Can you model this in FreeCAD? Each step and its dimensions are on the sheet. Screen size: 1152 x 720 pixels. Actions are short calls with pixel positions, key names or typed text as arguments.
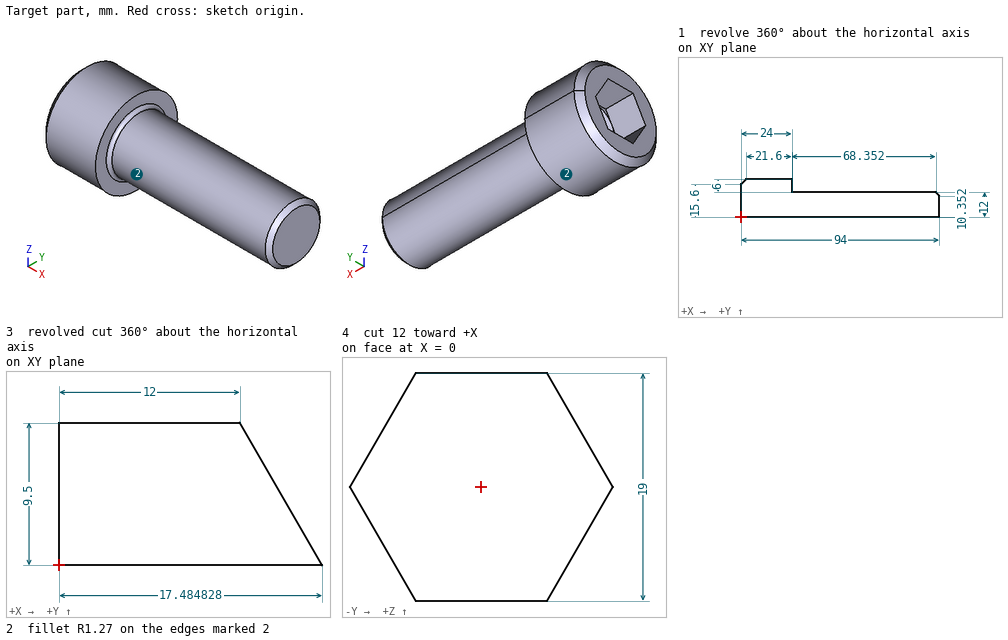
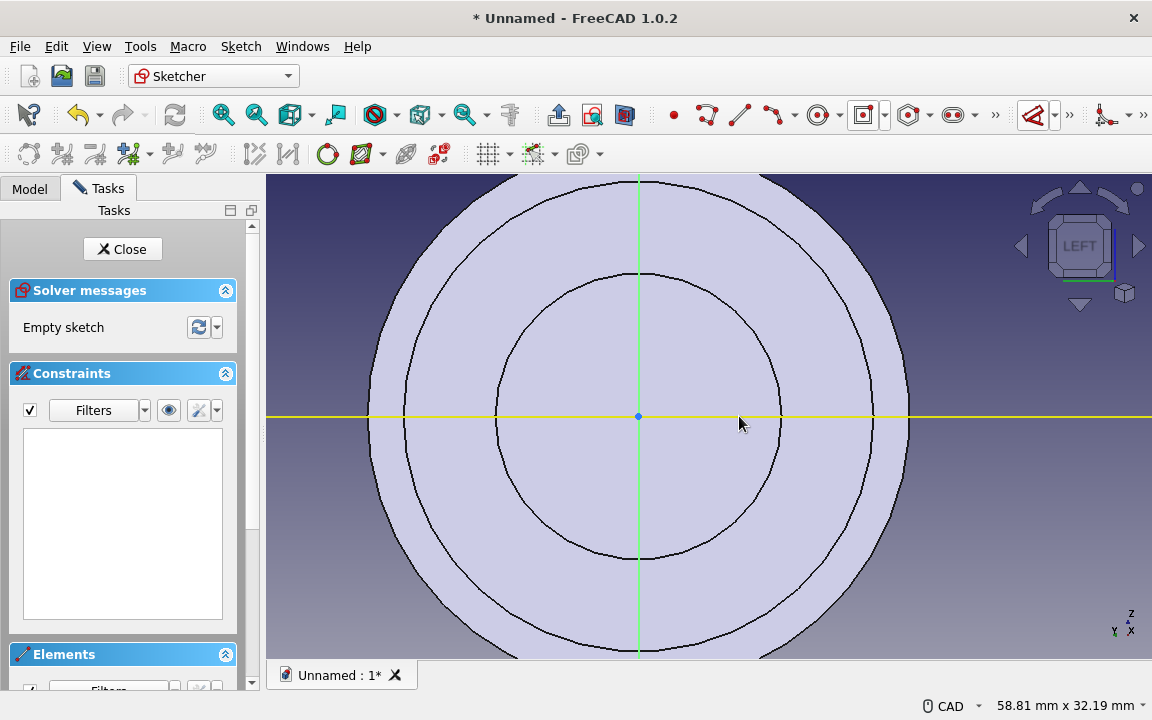
click(908, 116)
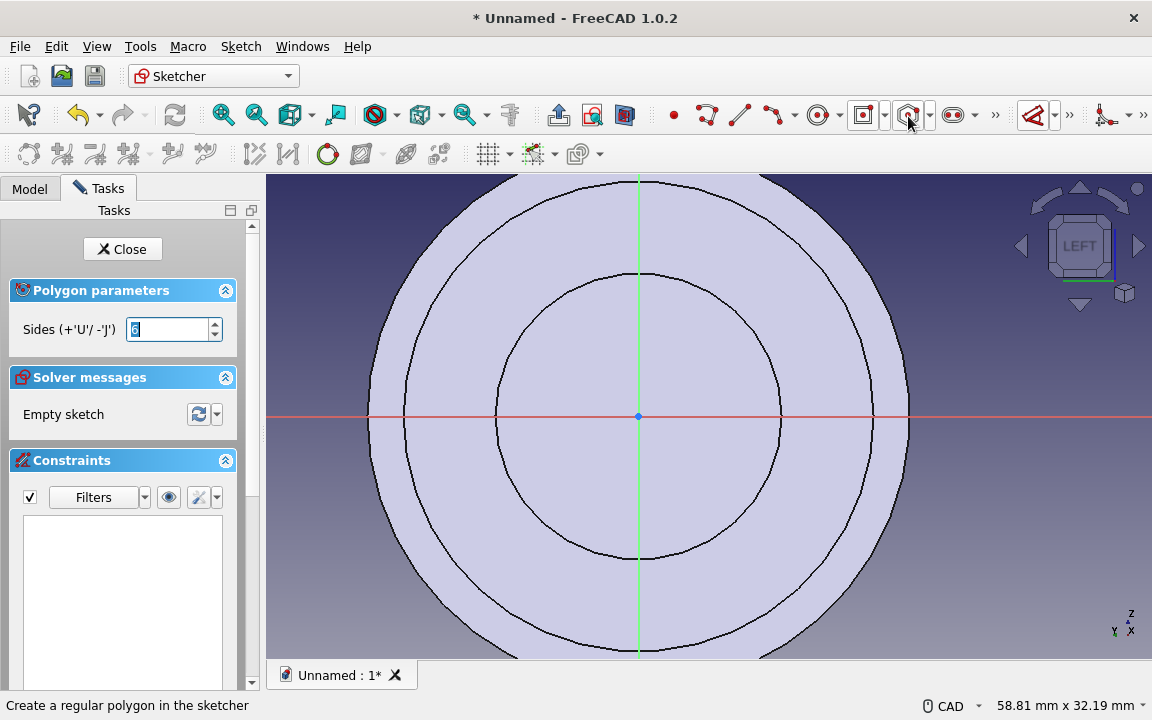
click(639, 416)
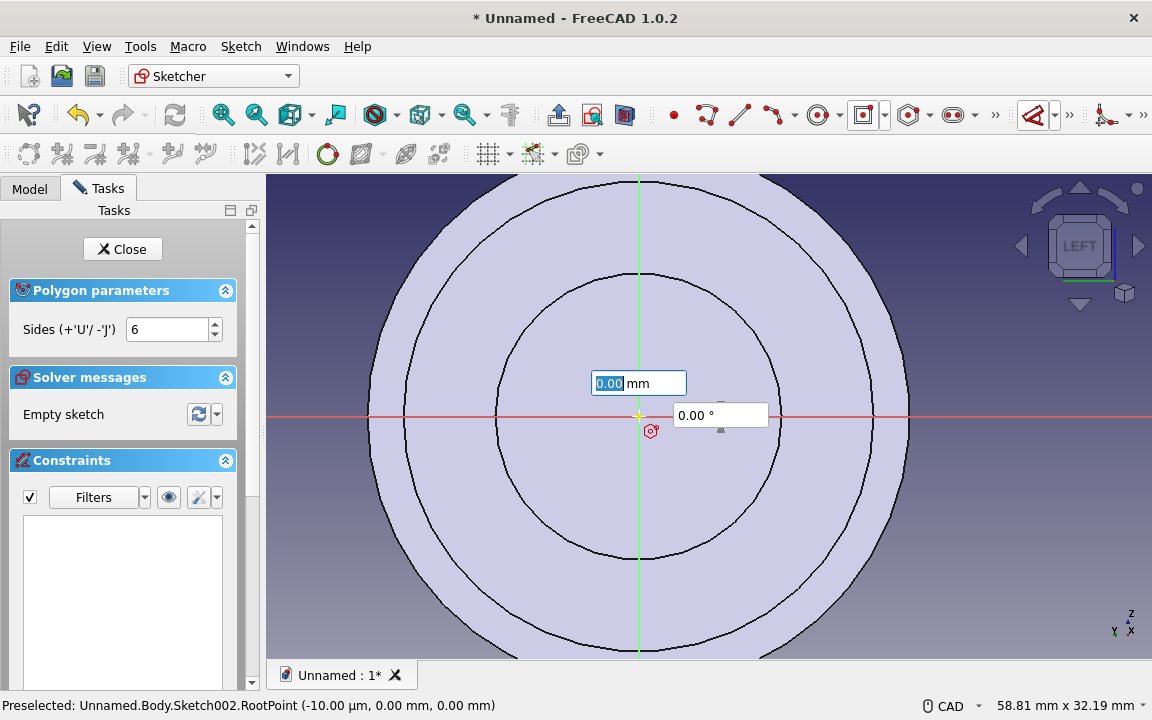
click(473, 416)
right_click(473, 416)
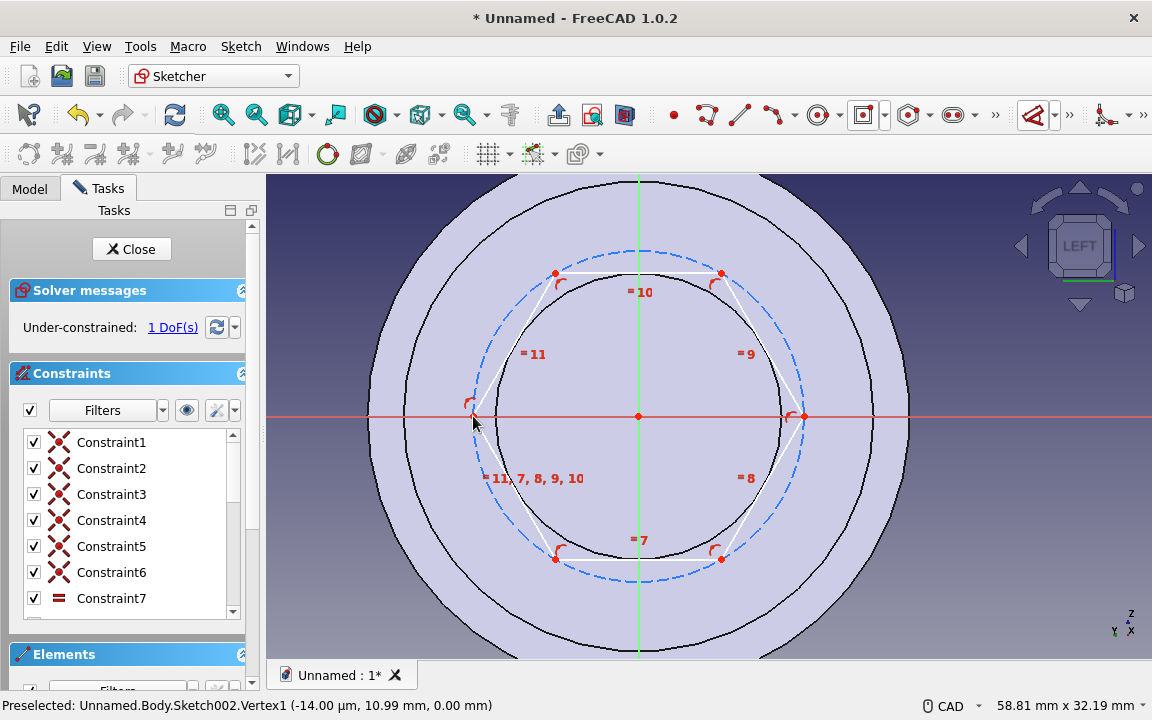
click(721, 560)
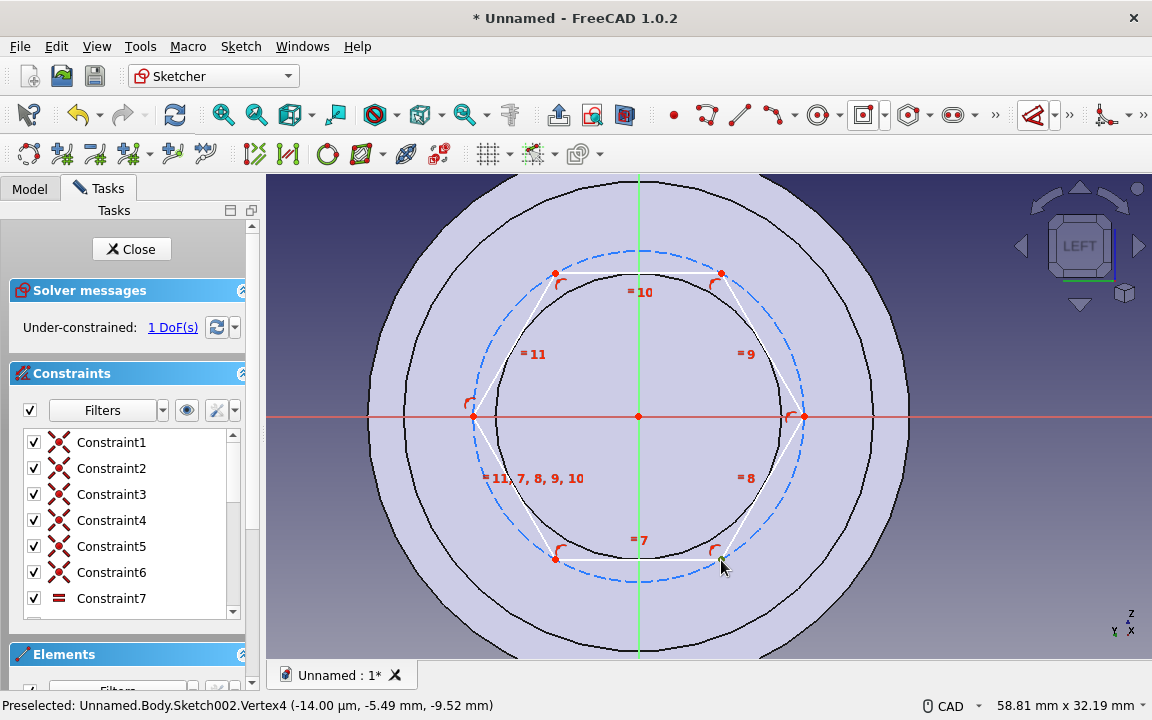
click(556, 273)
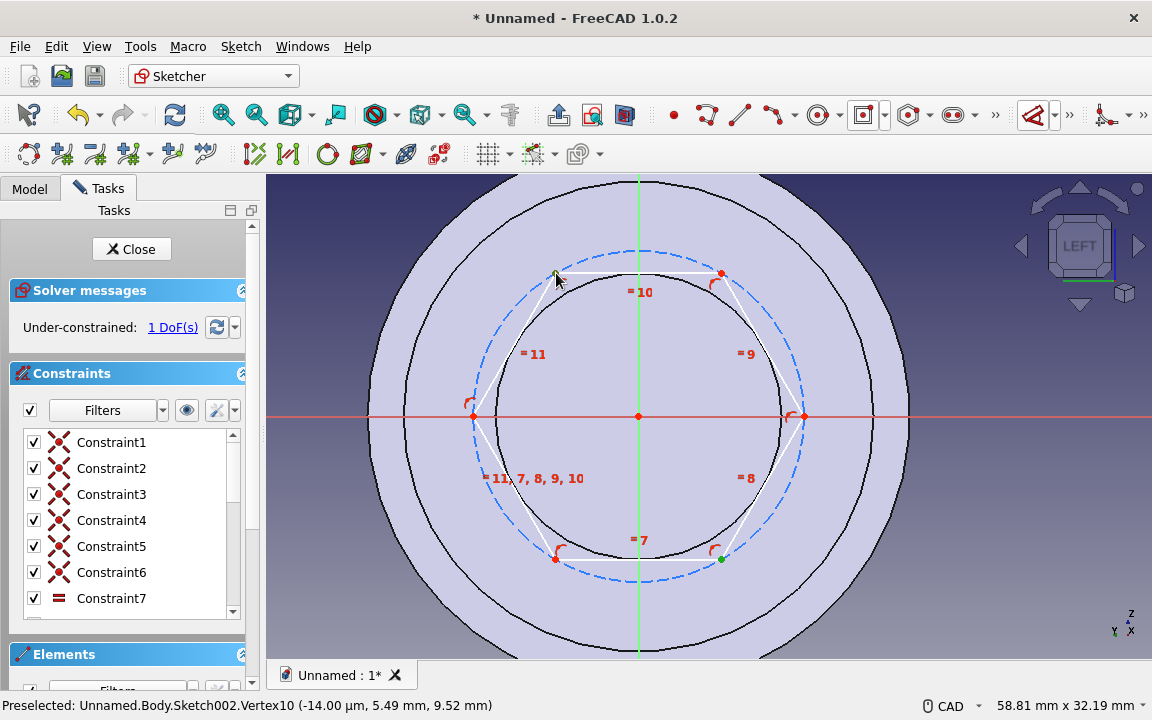
key(i)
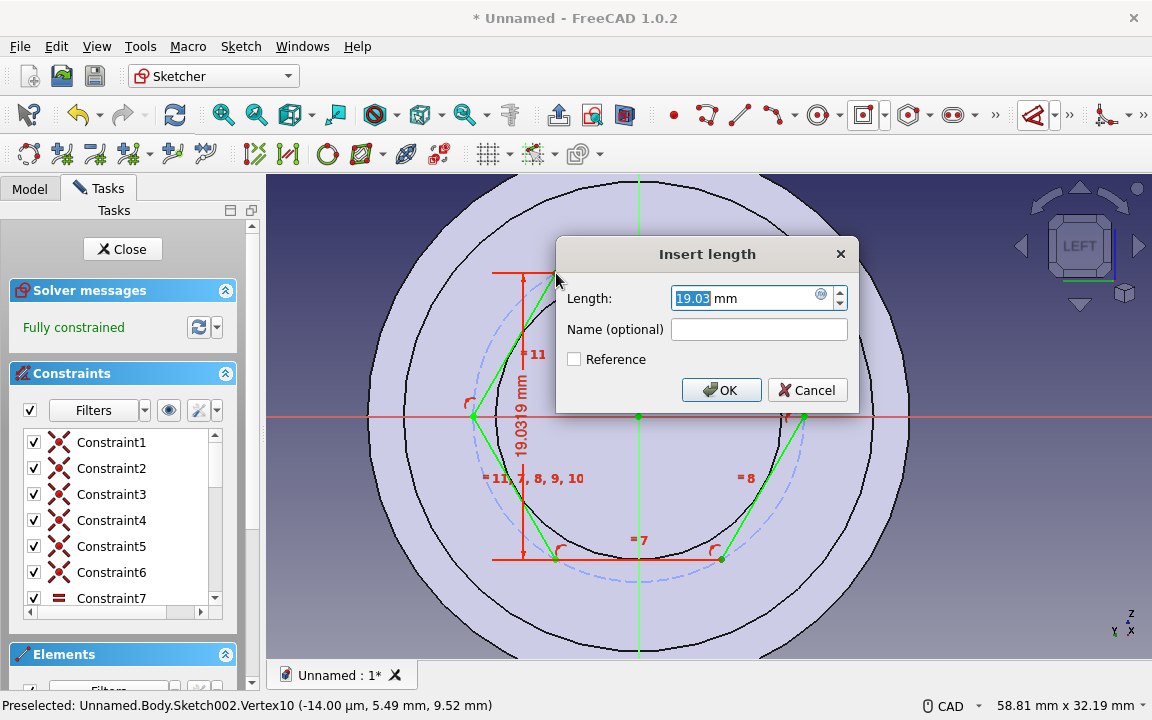
text(19)
key(Return)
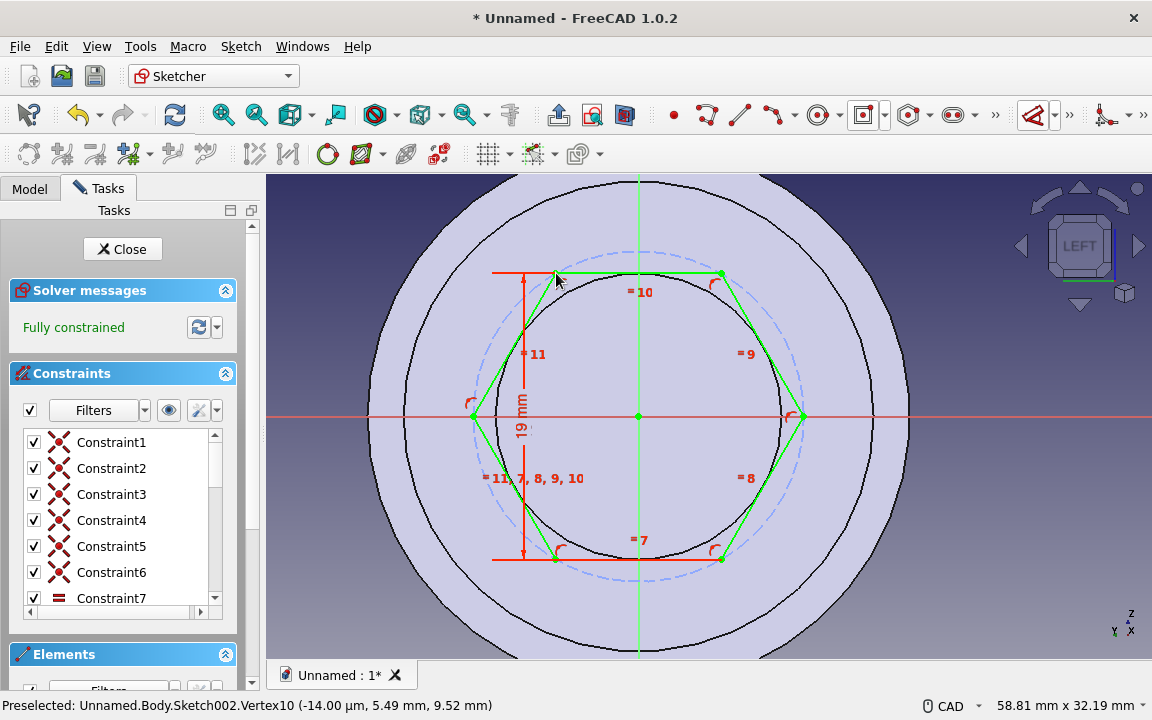
click(123, 249)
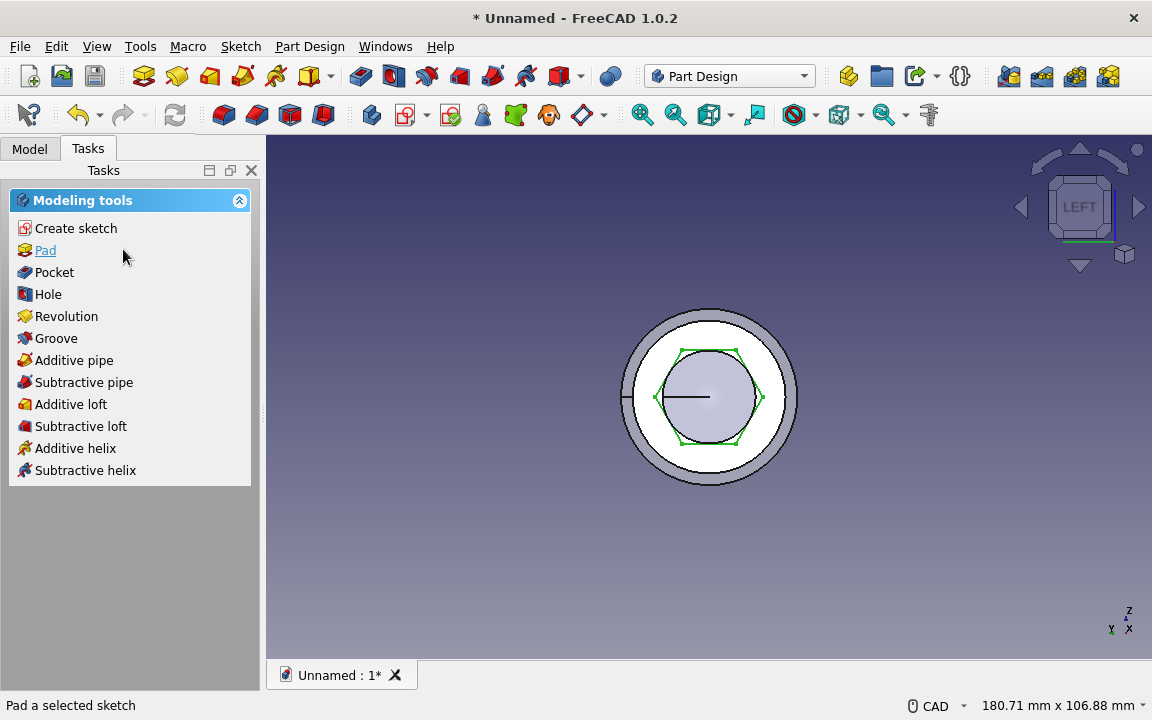
click(361, 76)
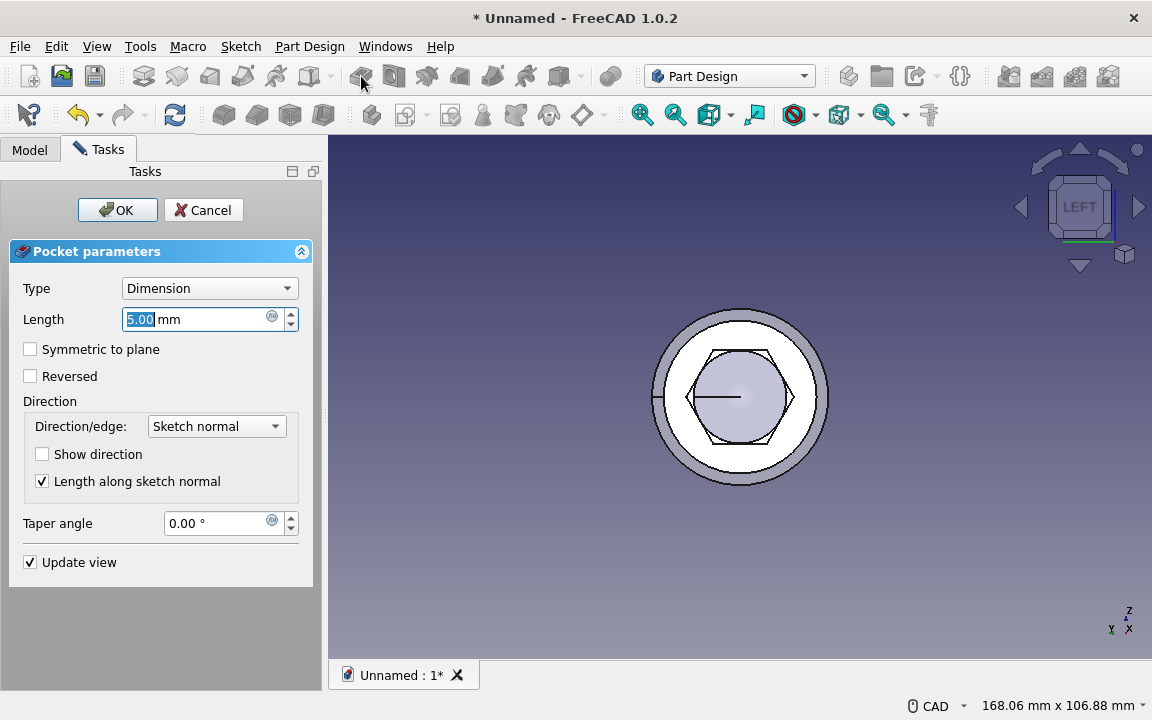
text(12)
key(Tab)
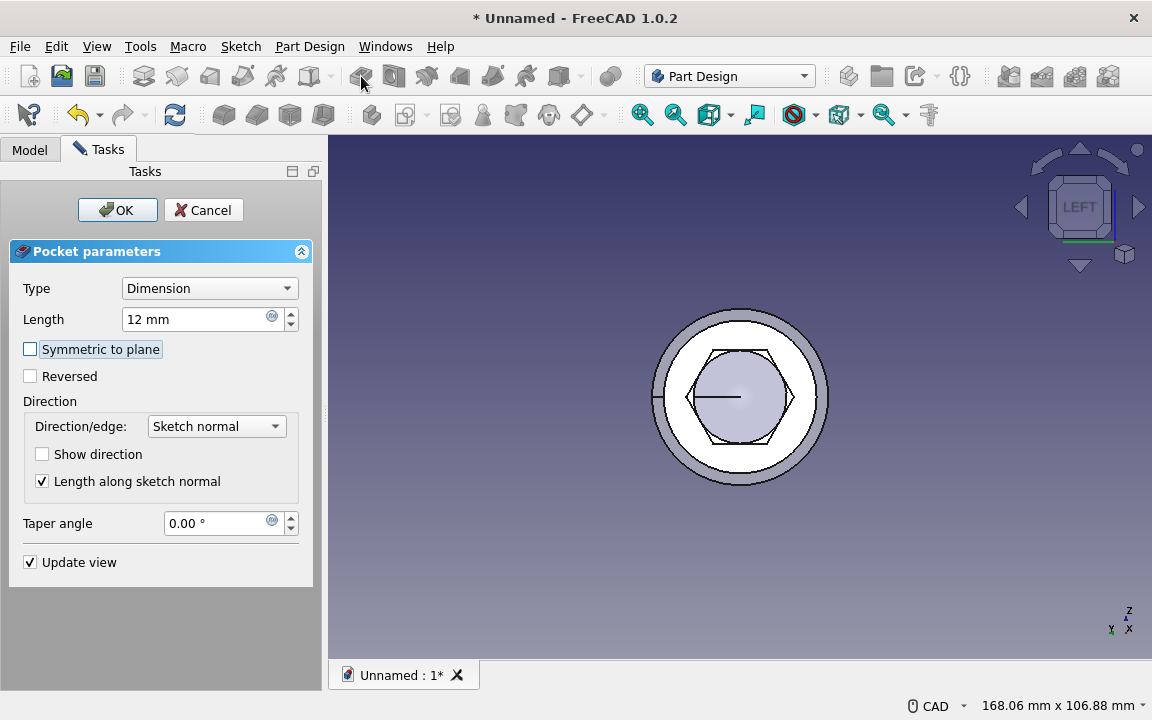
click(118, 210)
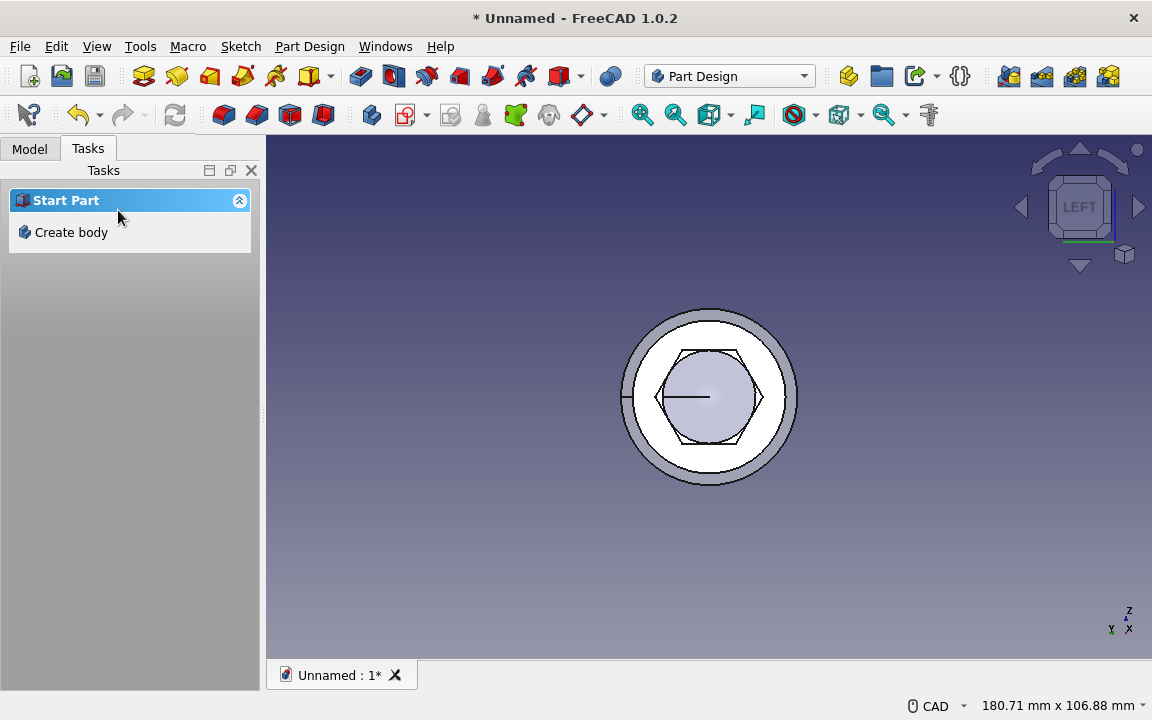
key(0)